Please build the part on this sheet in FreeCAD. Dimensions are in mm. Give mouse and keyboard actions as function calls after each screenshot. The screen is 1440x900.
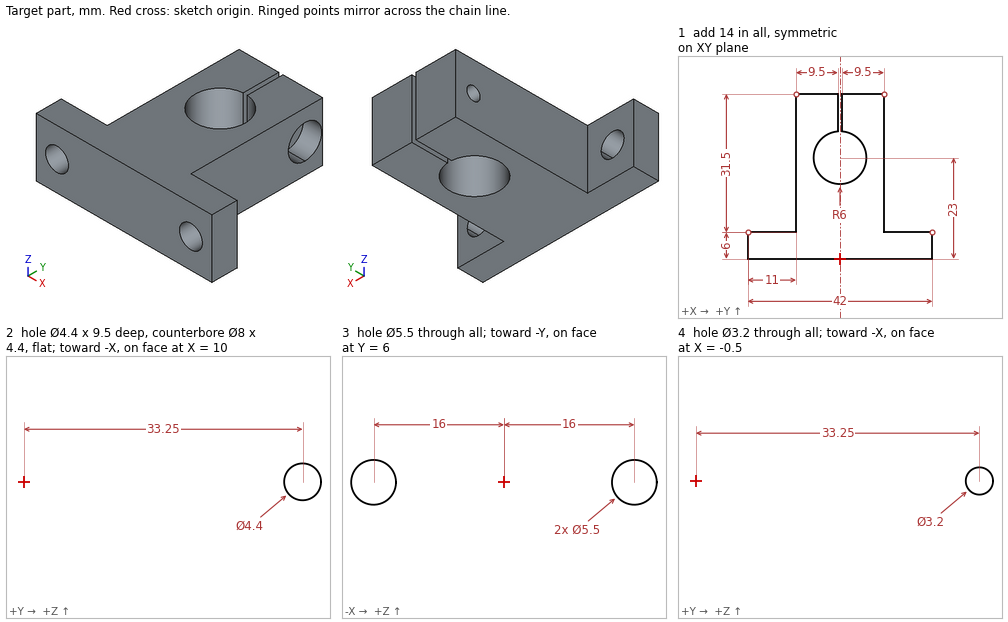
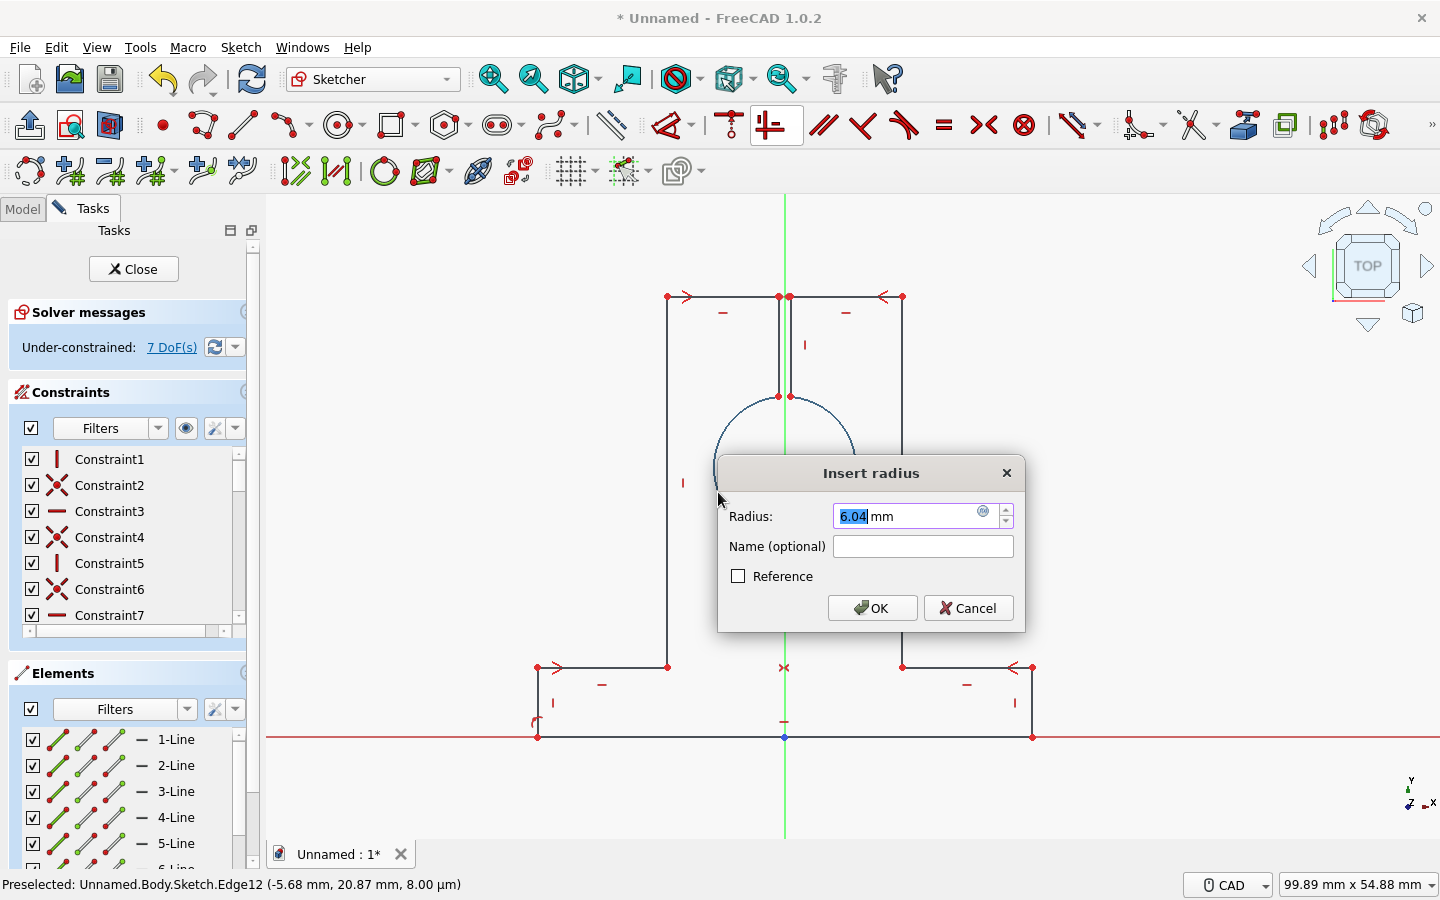
text(6)
key(Return)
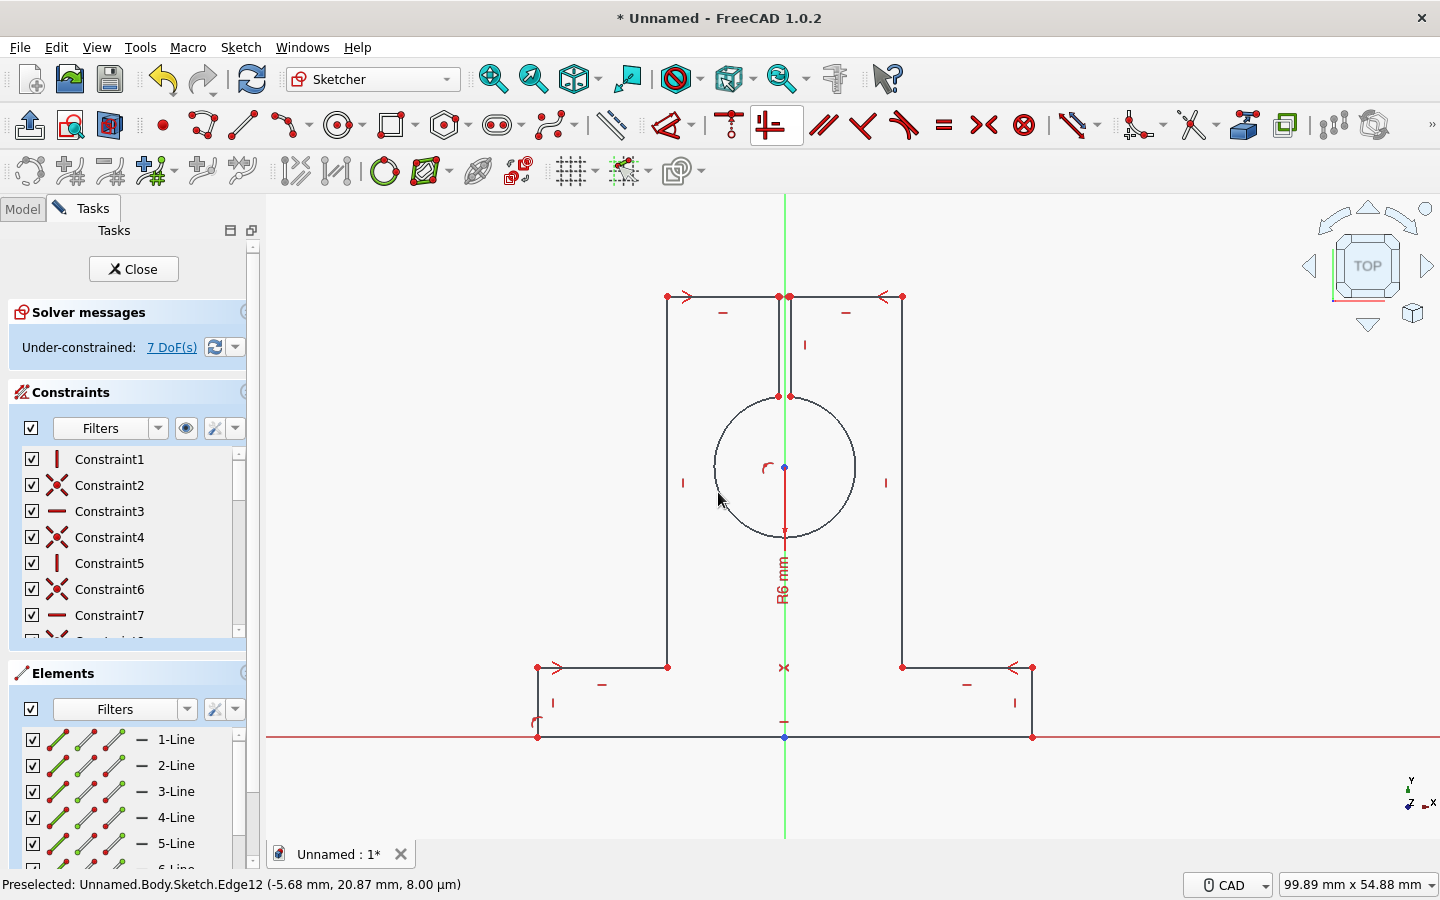
click(538, 689)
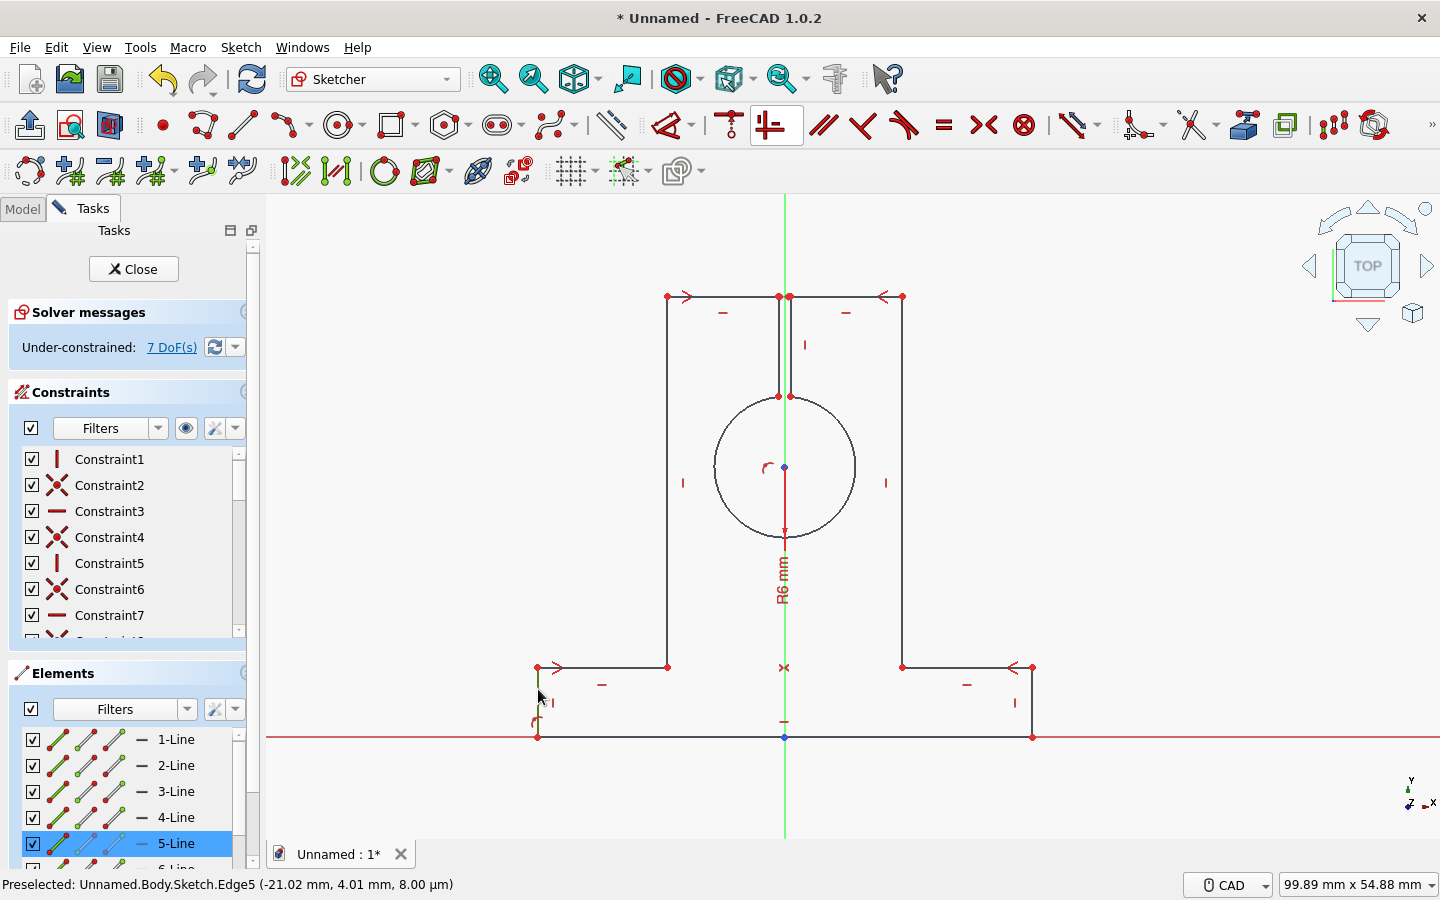
click(694, 126)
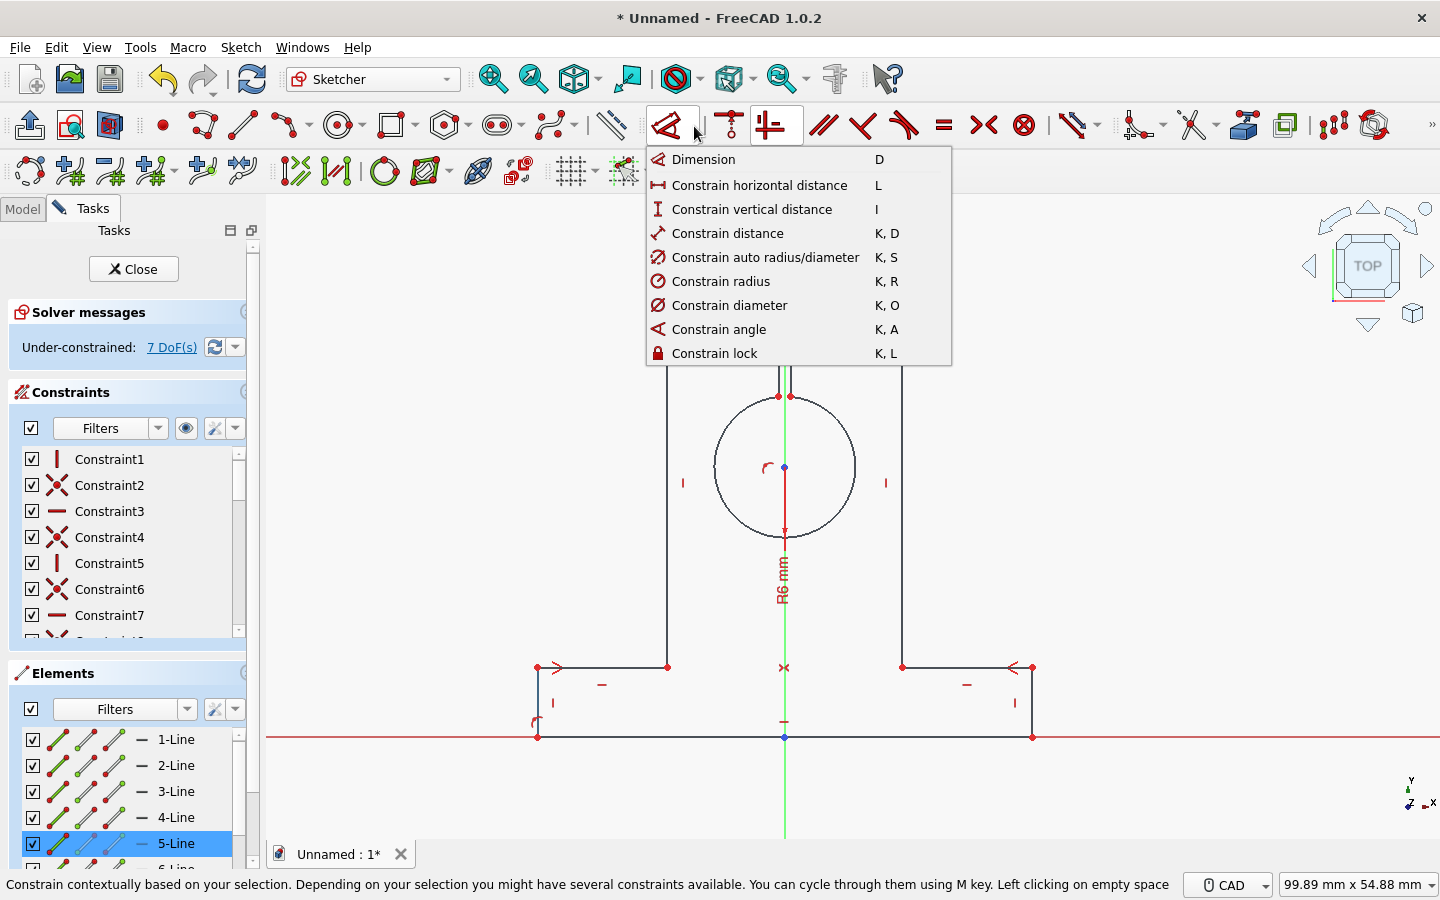
click(799, 209)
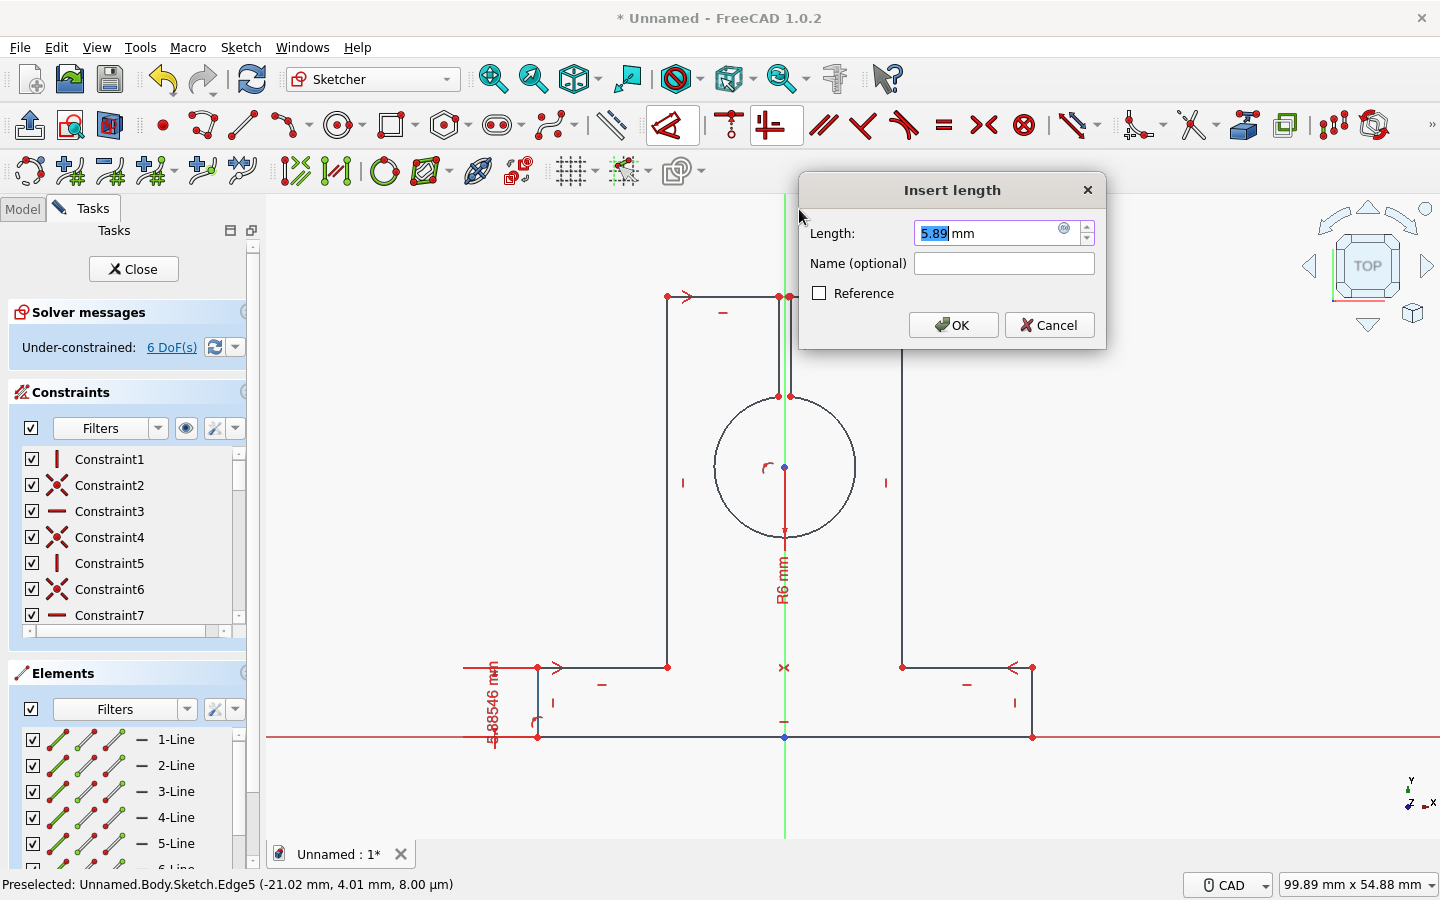
text(6)
key(Return)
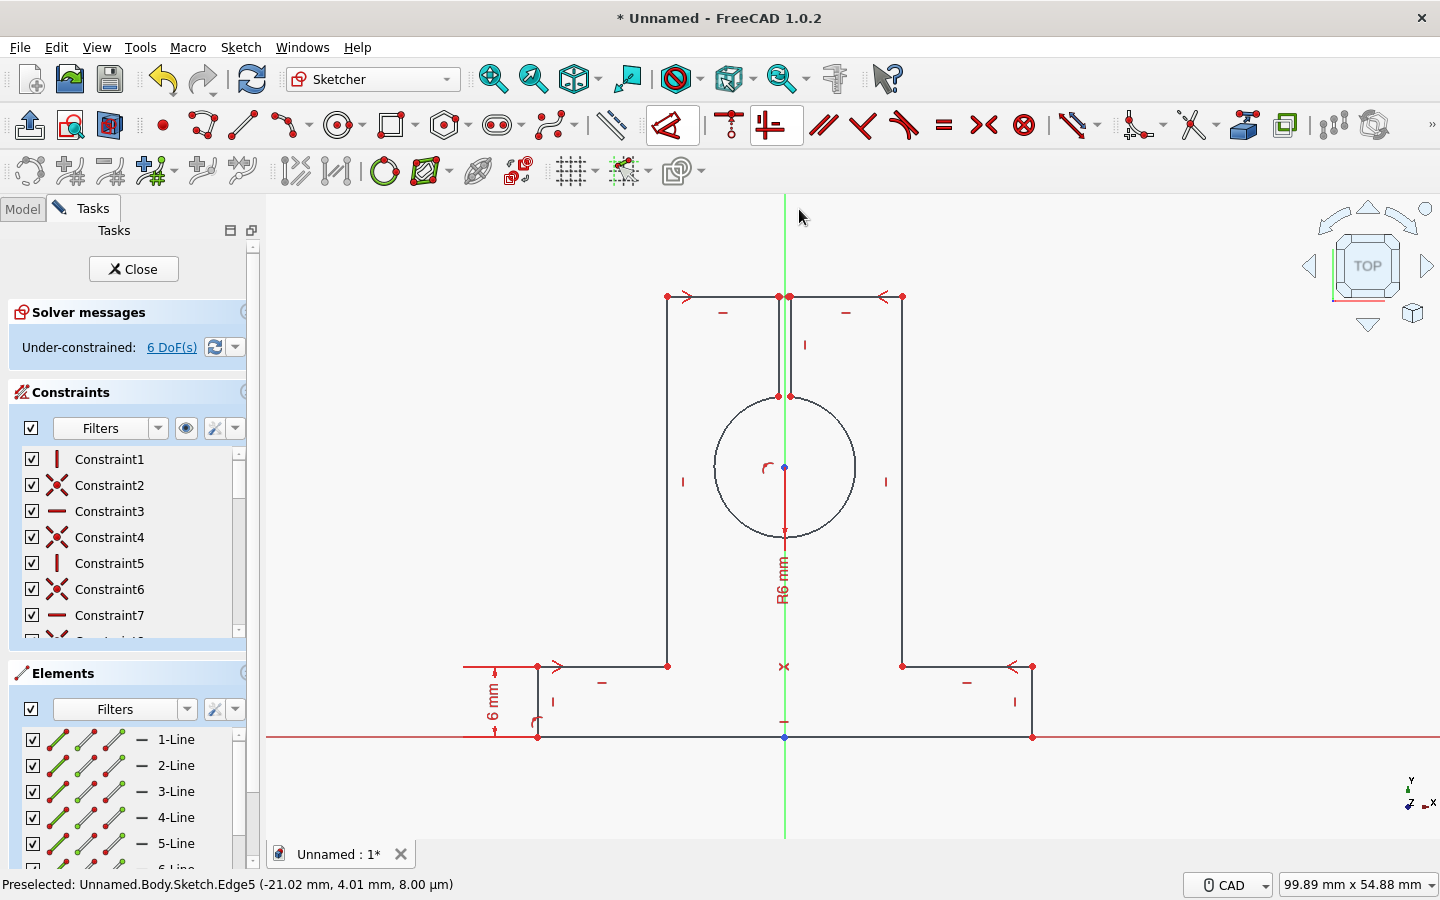
click(629, 667)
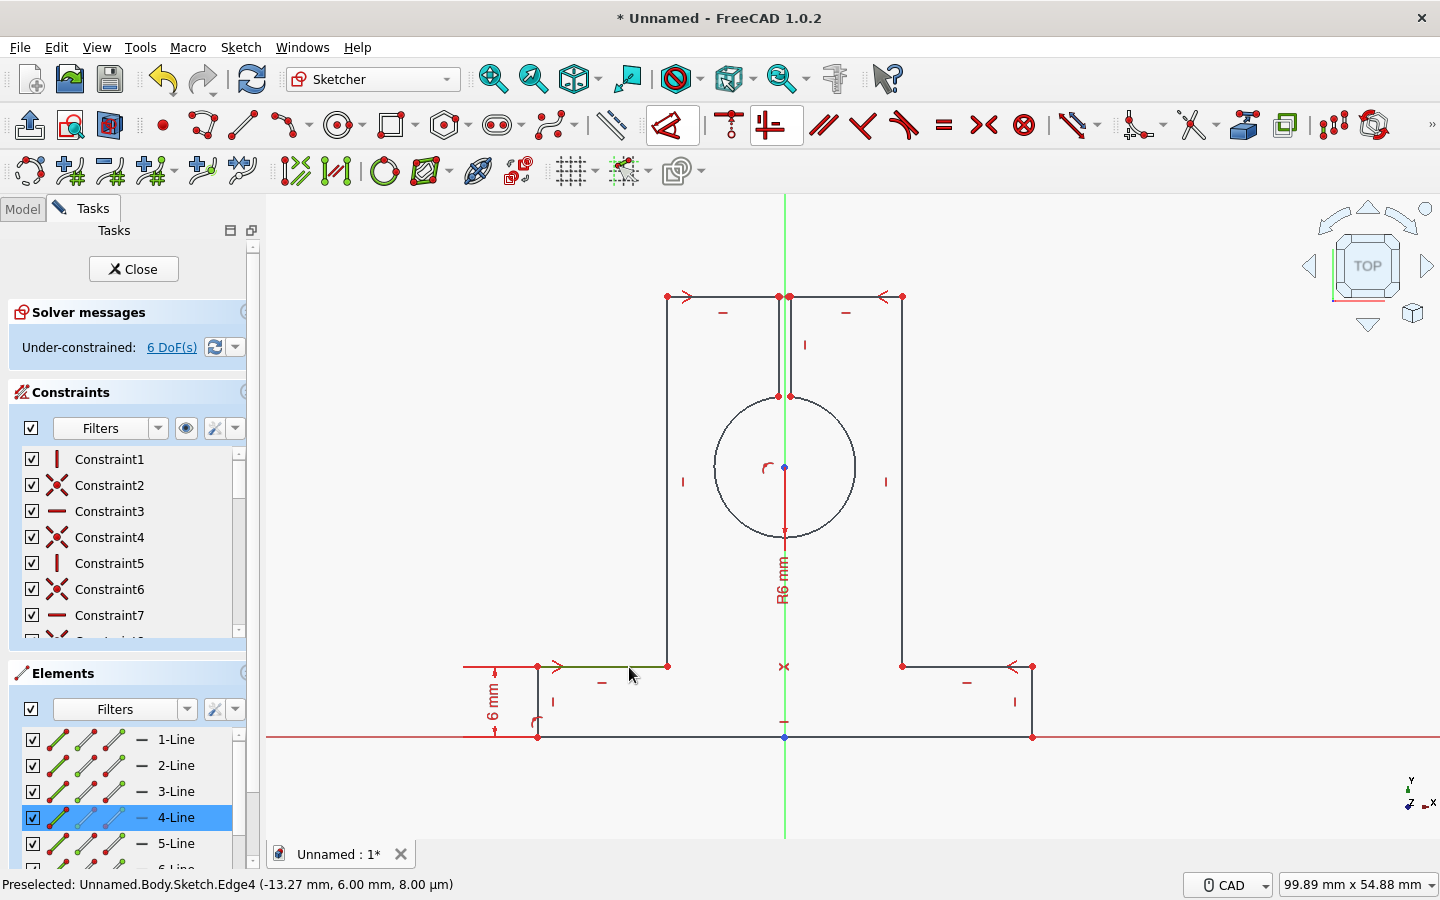
key(l)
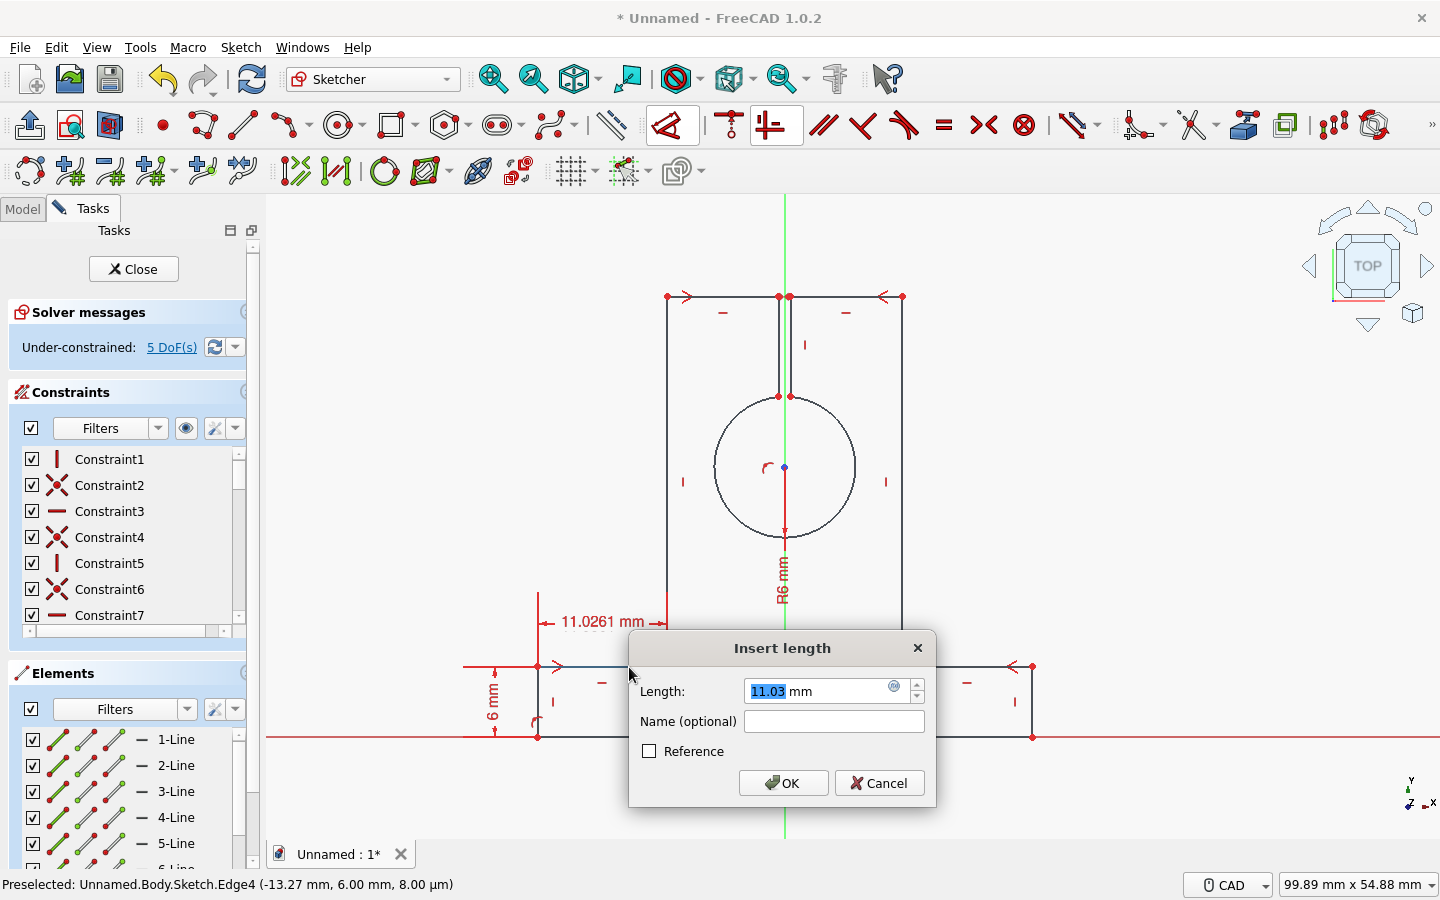
text(11)
key(Return)